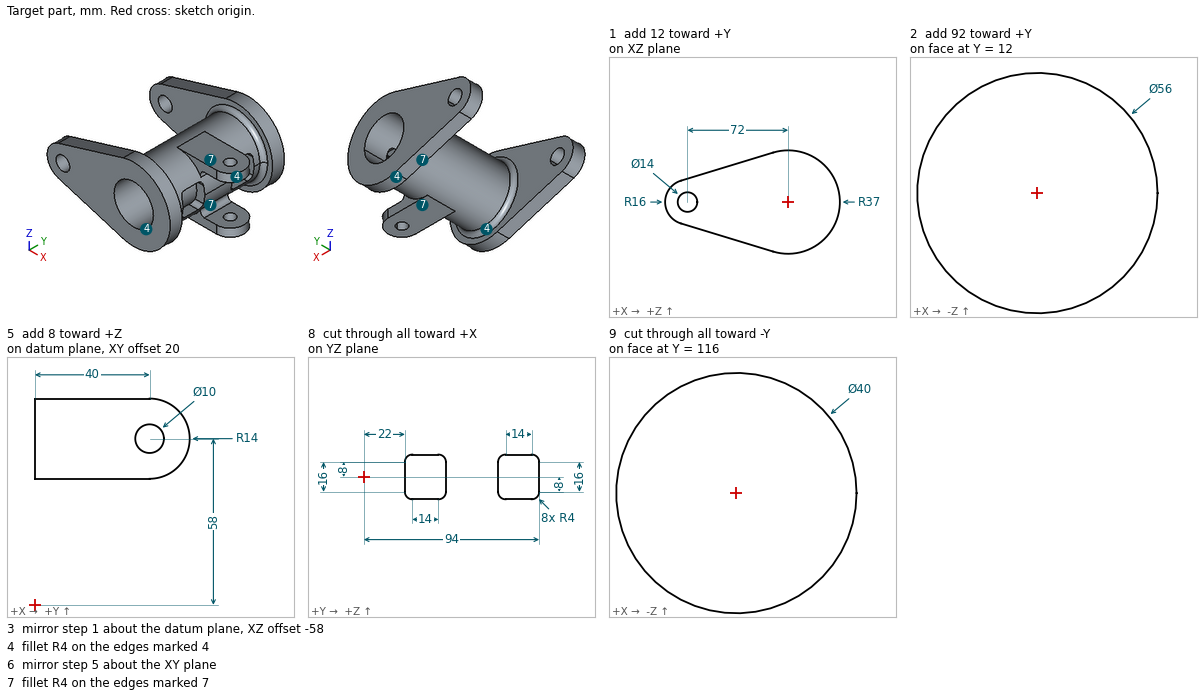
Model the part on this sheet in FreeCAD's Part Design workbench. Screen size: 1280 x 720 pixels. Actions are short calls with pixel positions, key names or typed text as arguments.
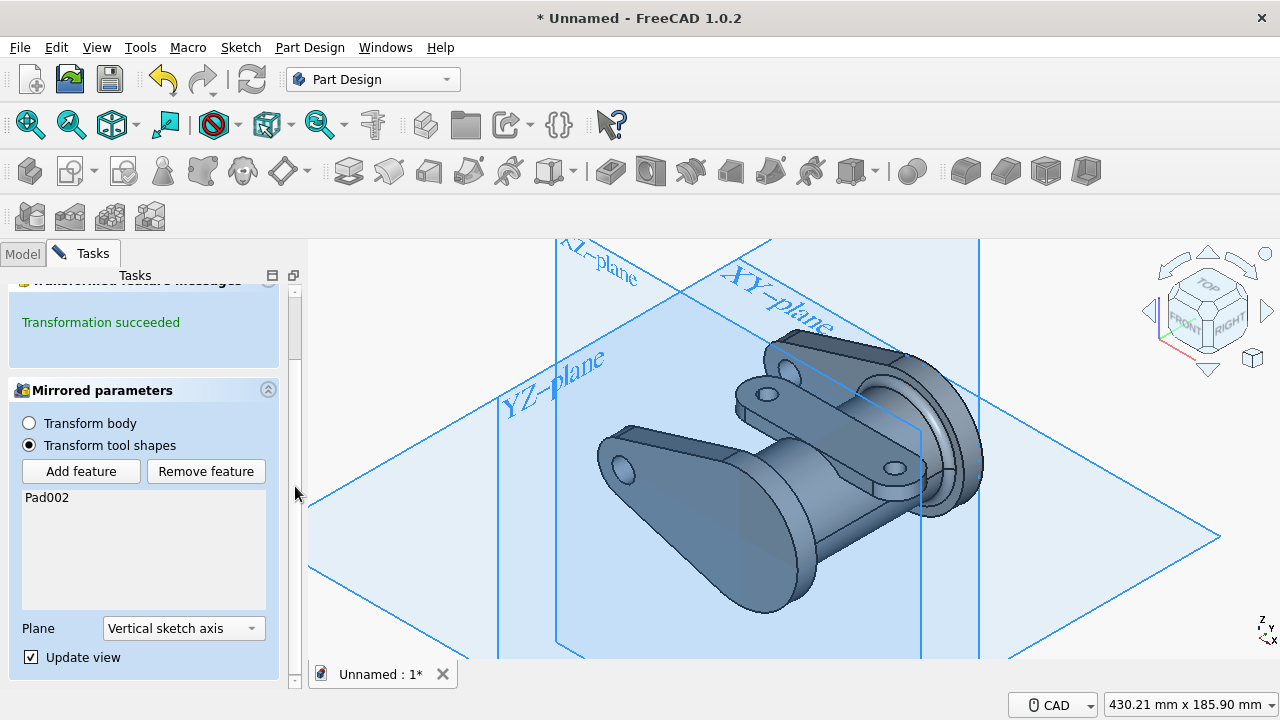
click(184, 628)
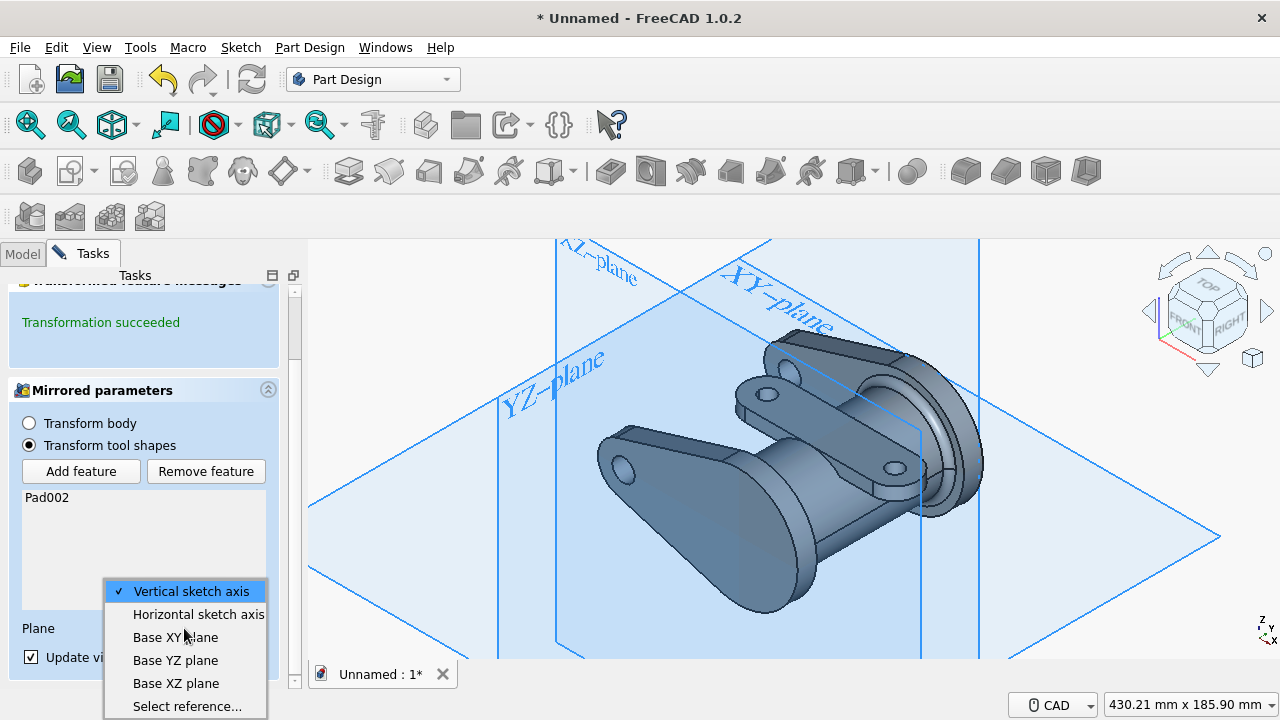
click(184, 638)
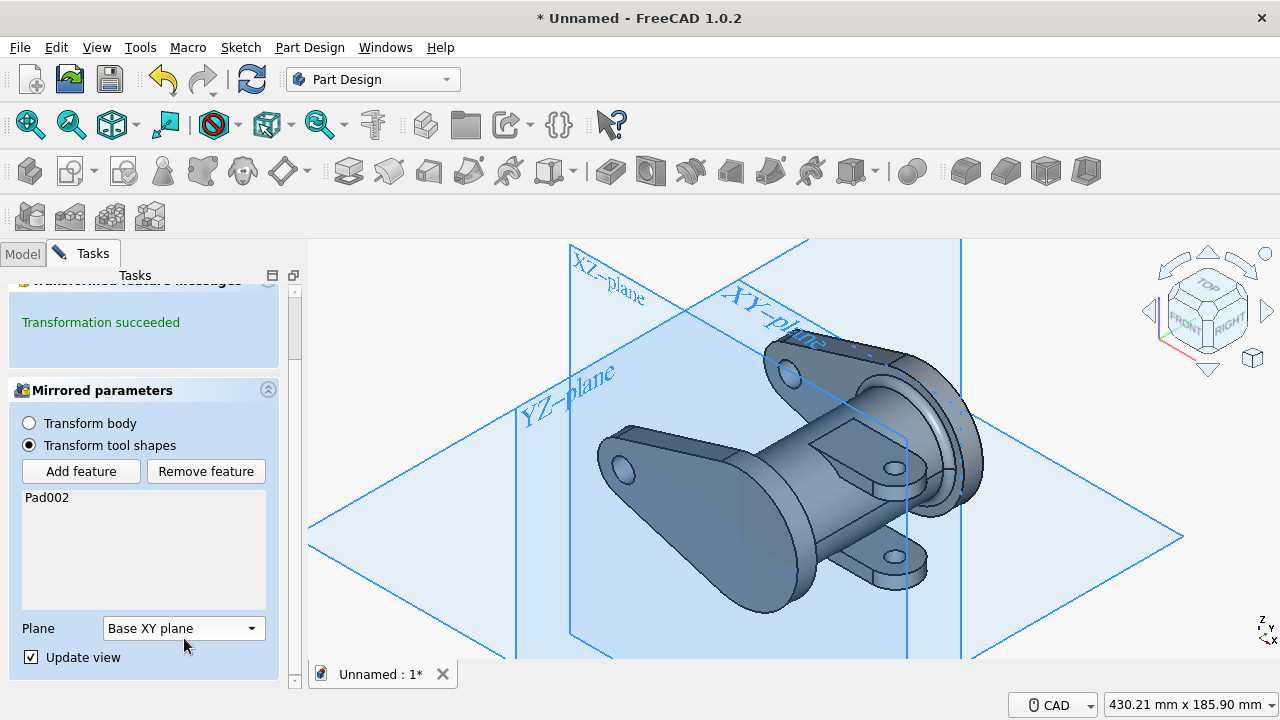
scroll(295, 486, up, 3)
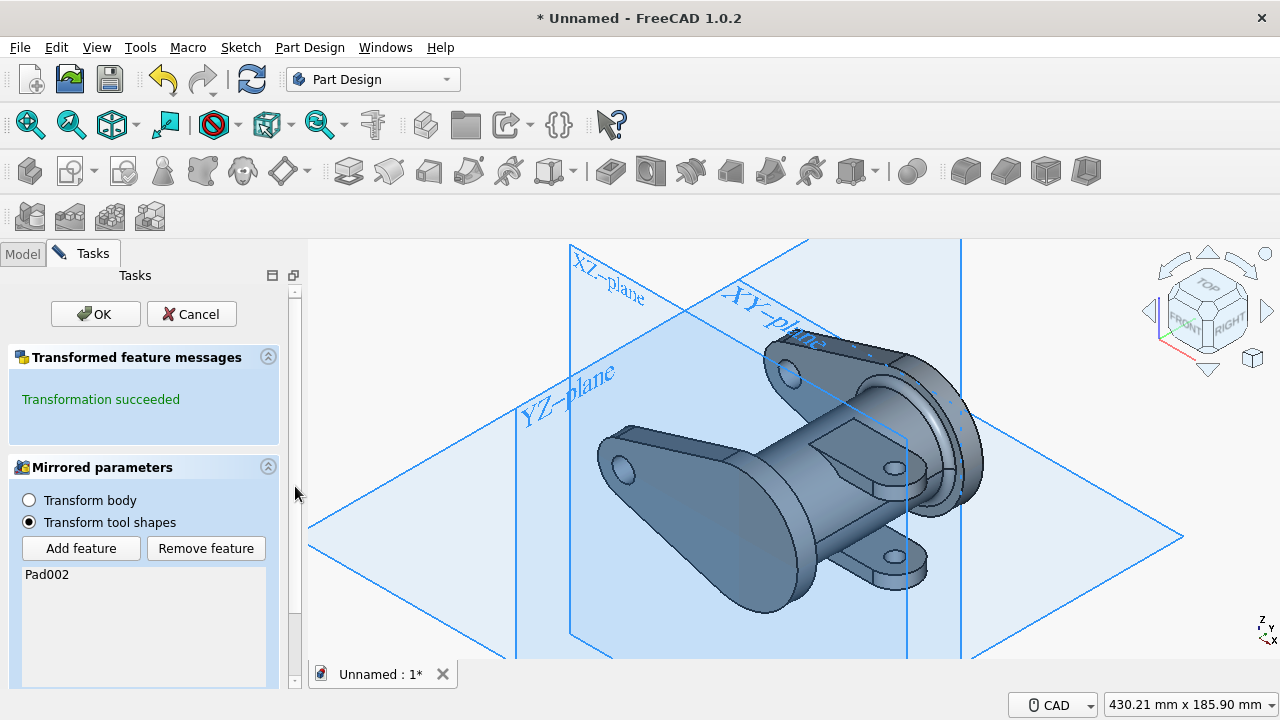
click(96, 314)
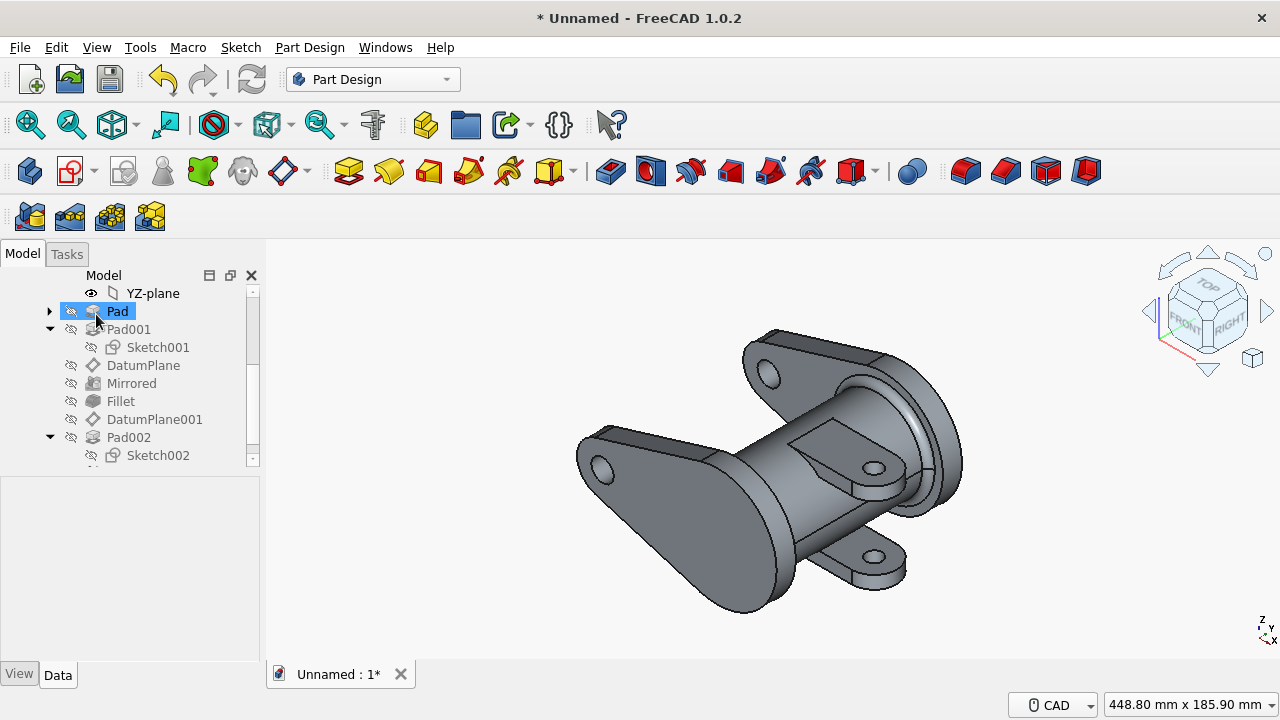
key(2)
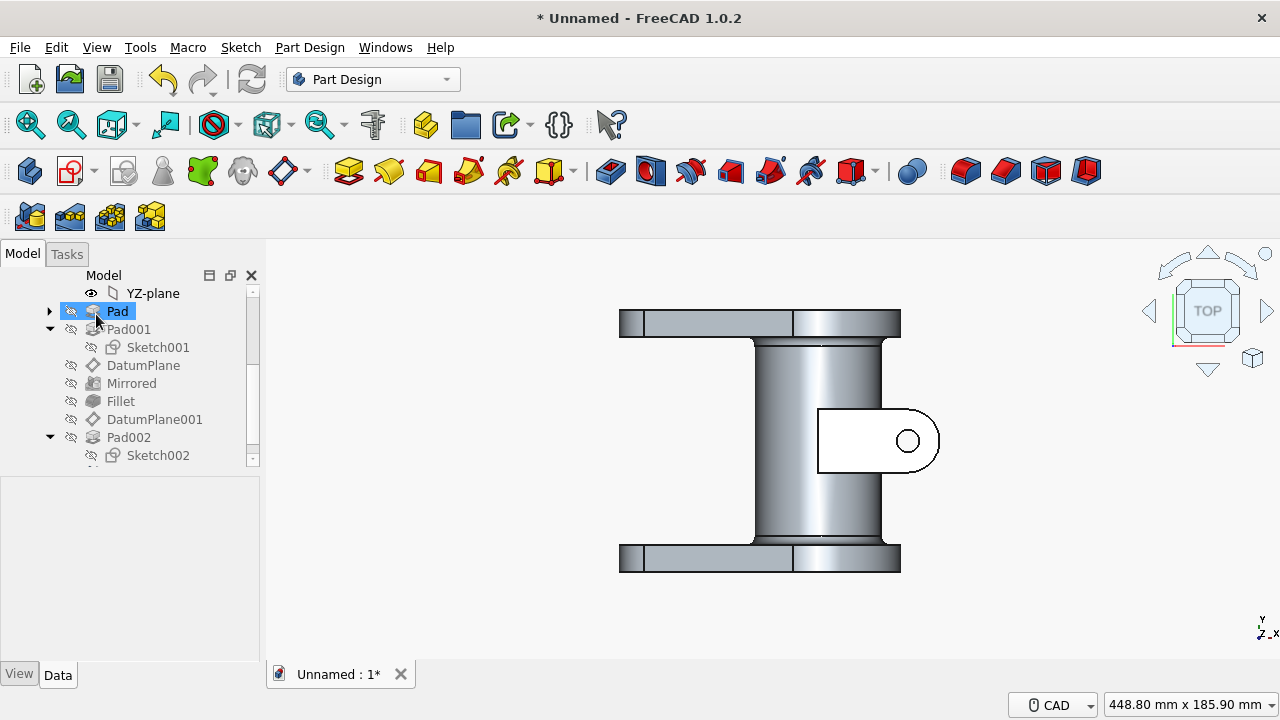
key(0)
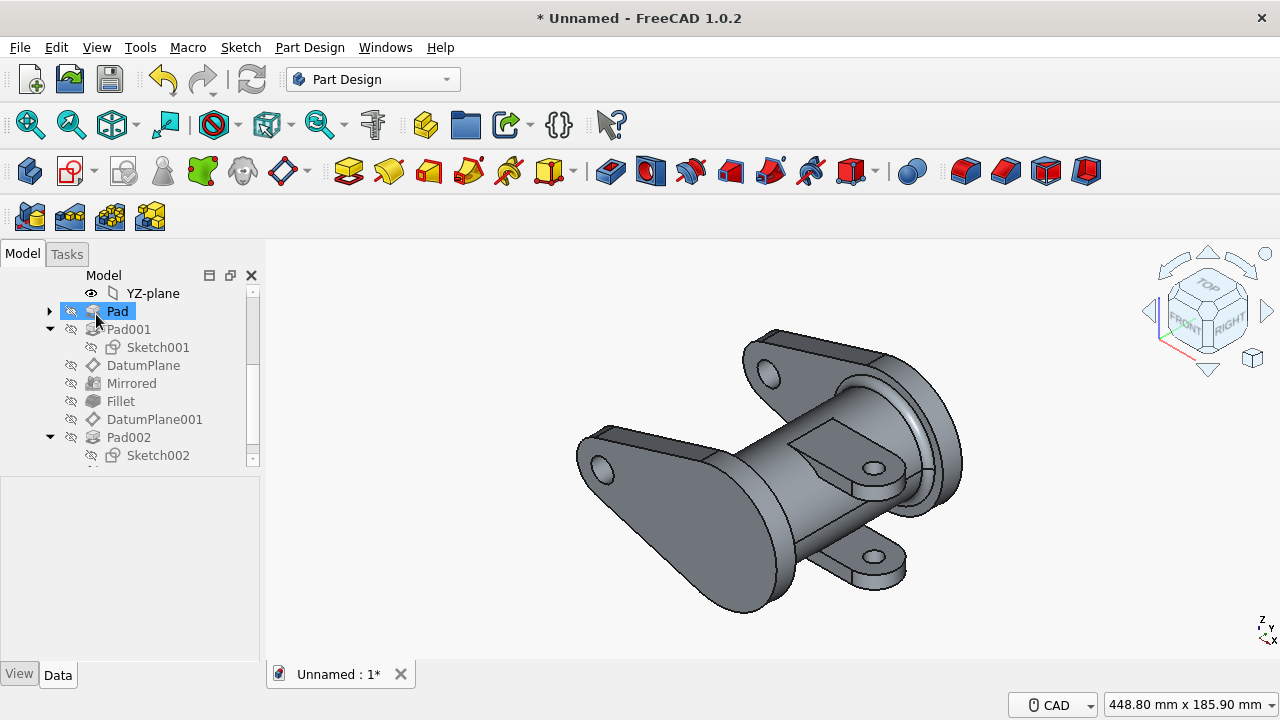
key(1)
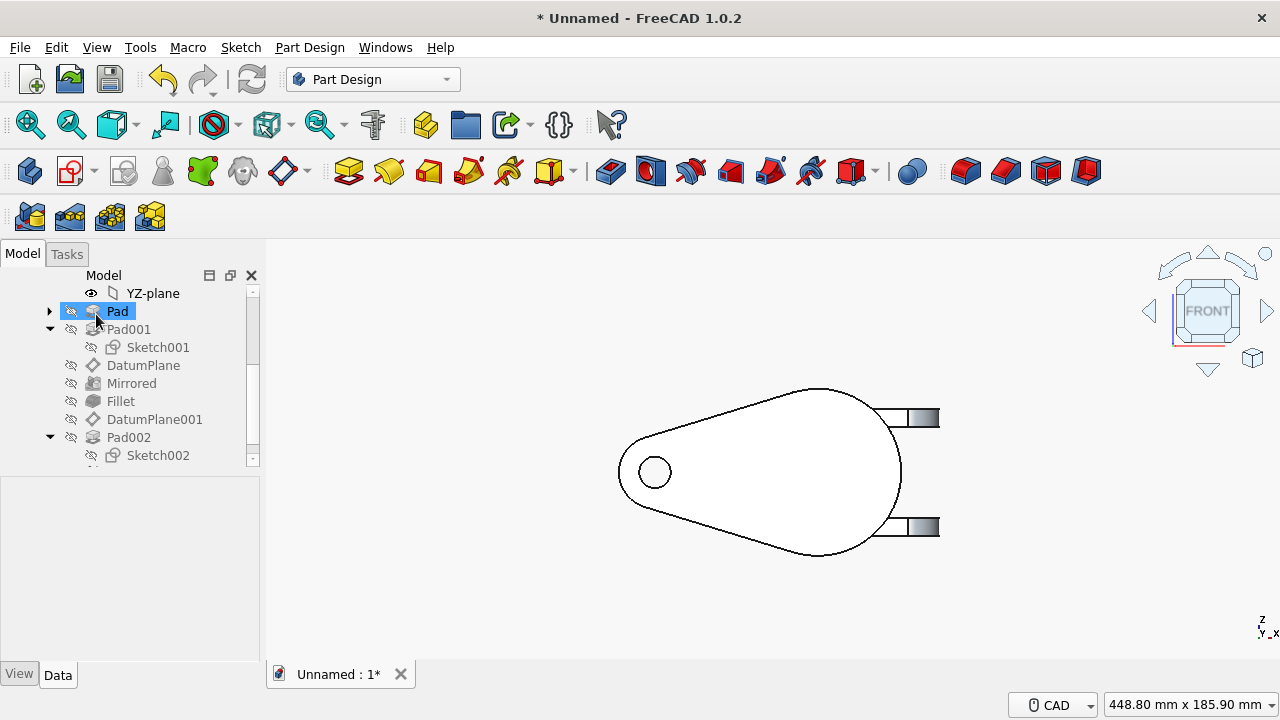
click(32, 126)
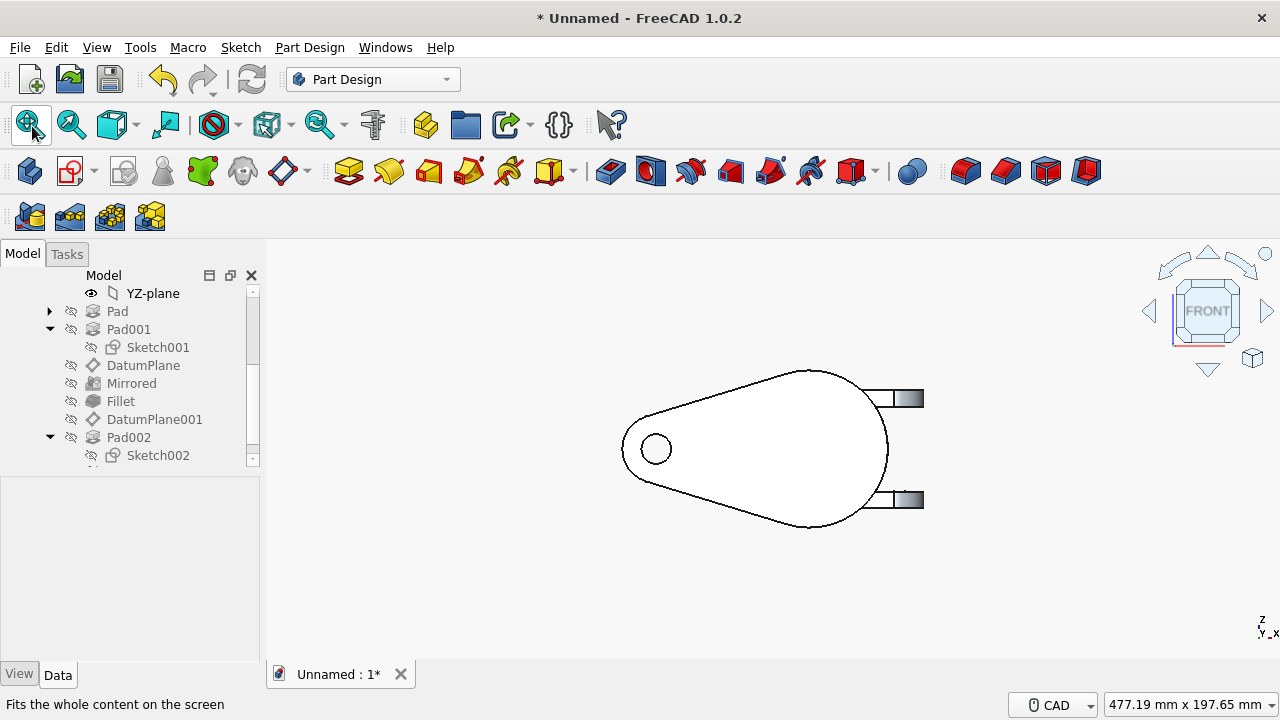
key(3)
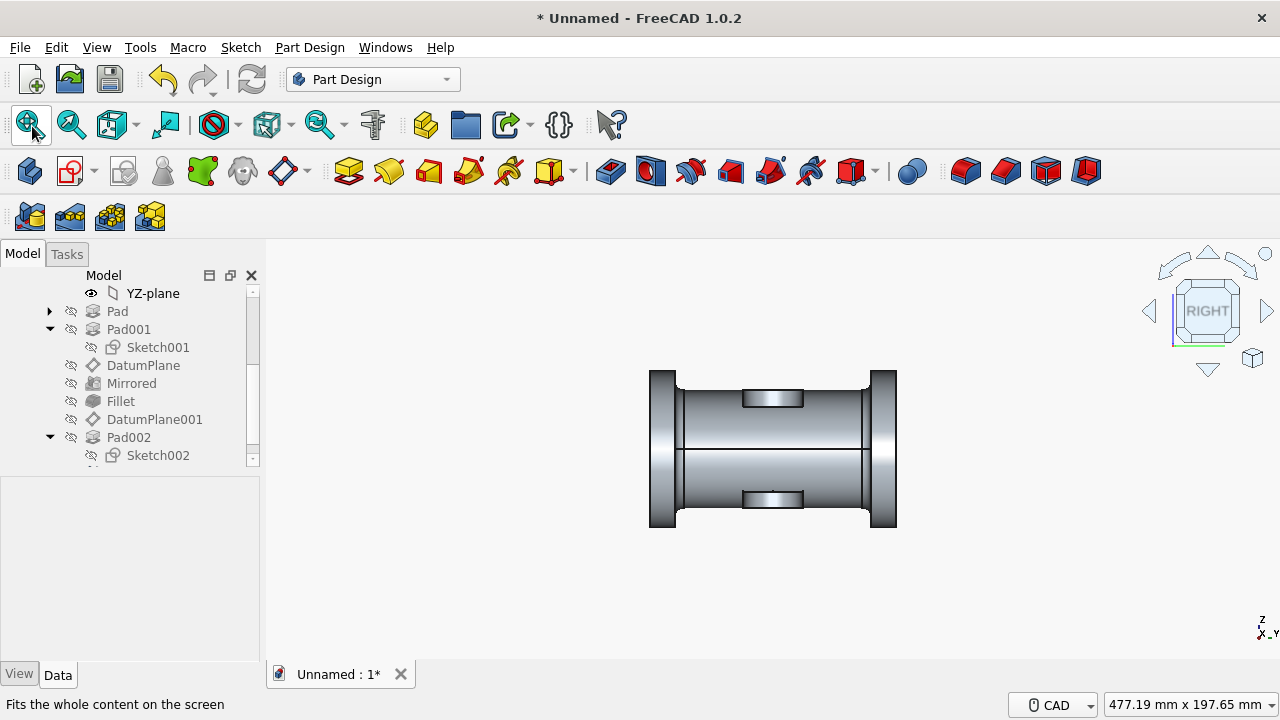
click(32, 126)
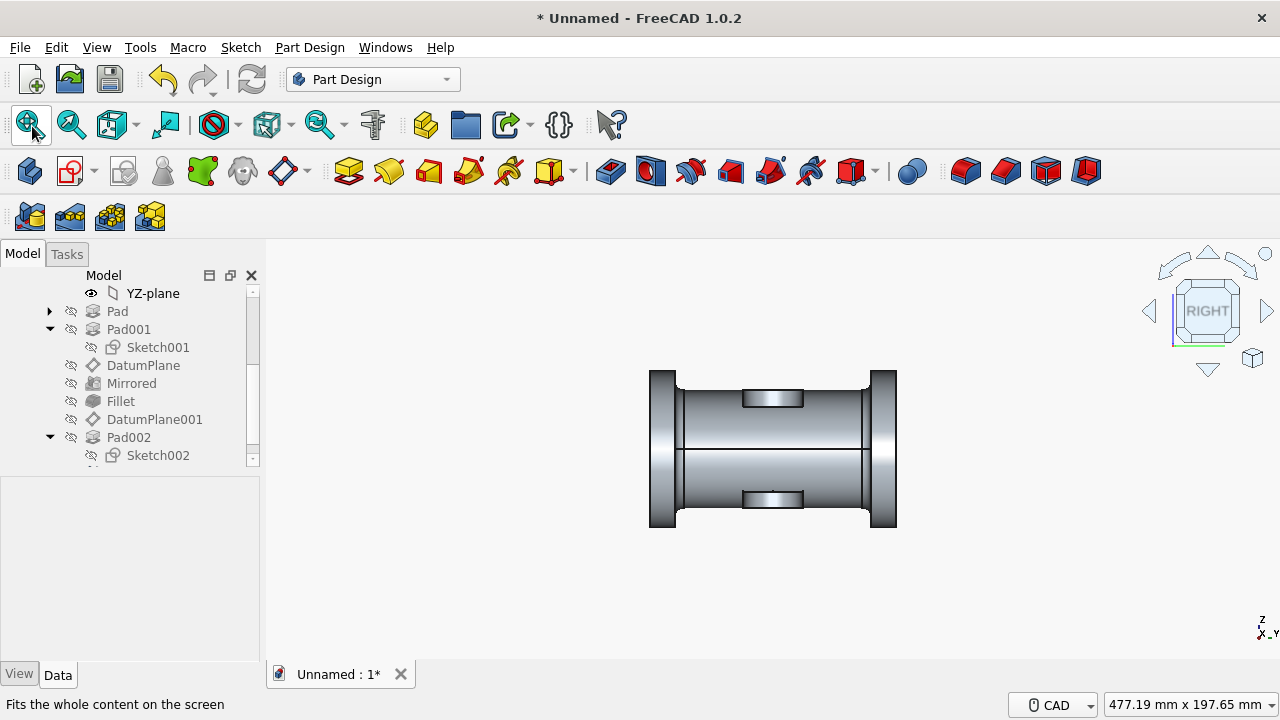
key(5)